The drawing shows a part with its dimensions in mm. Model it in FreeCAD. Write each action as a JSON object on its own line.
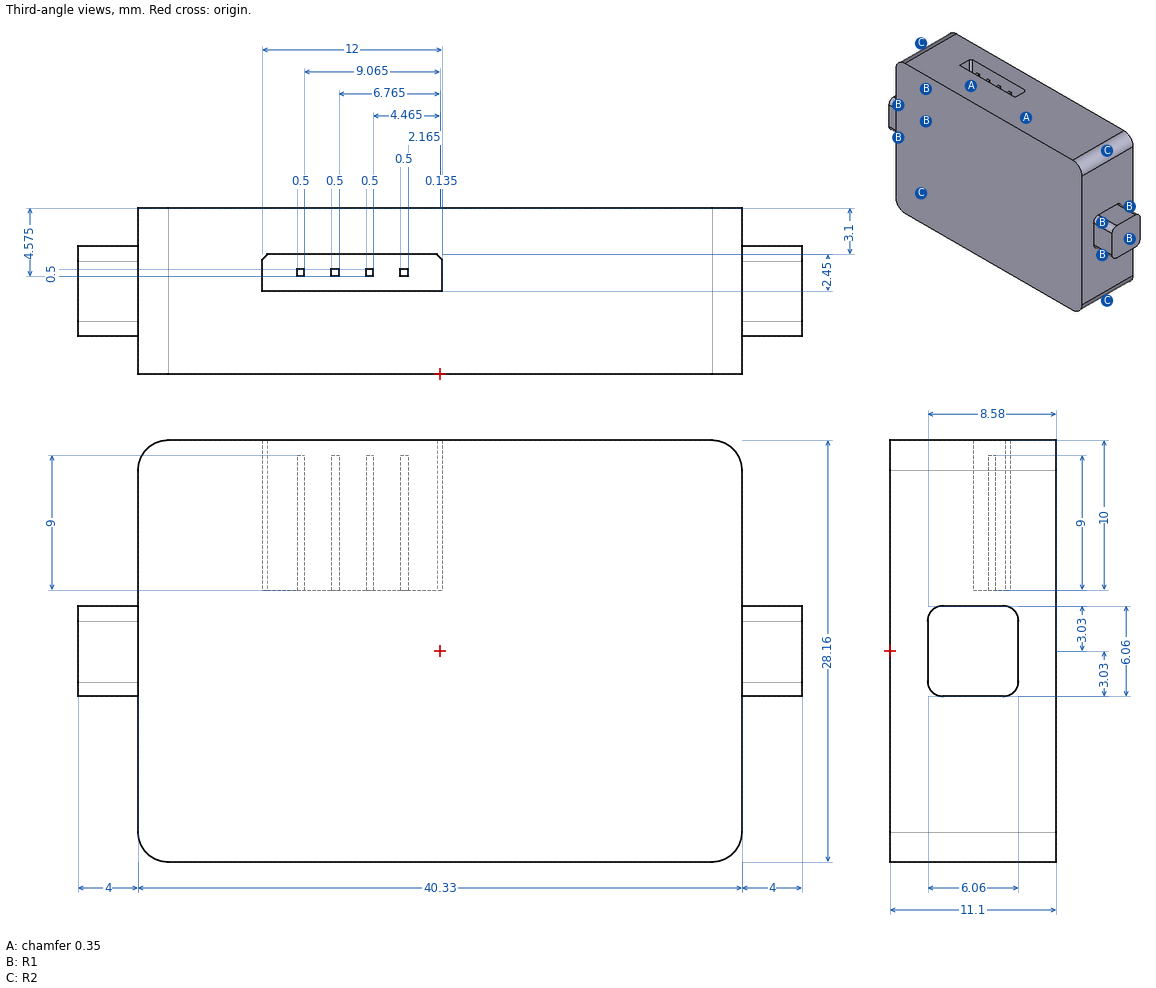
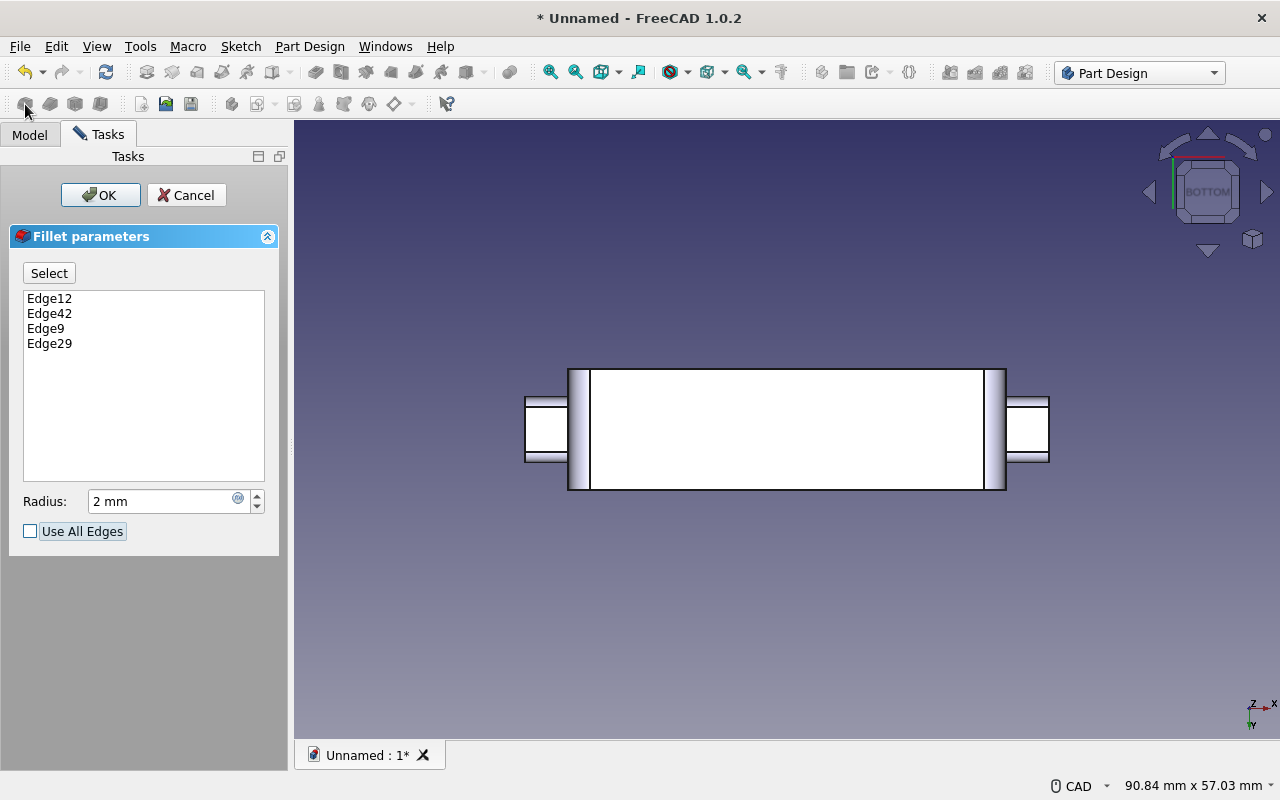
{"action": "left_click", "coordinate": [101, 195]}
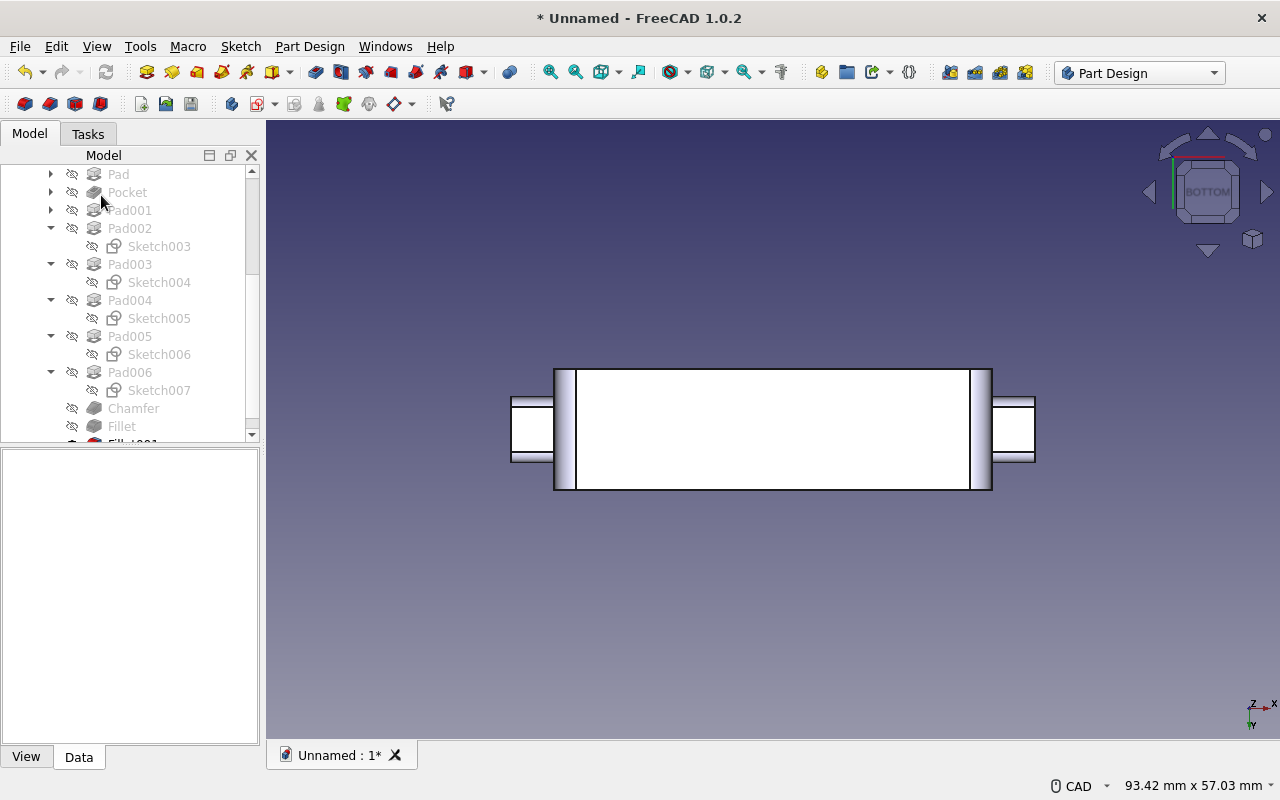
{"action": "key", "text": "0"}